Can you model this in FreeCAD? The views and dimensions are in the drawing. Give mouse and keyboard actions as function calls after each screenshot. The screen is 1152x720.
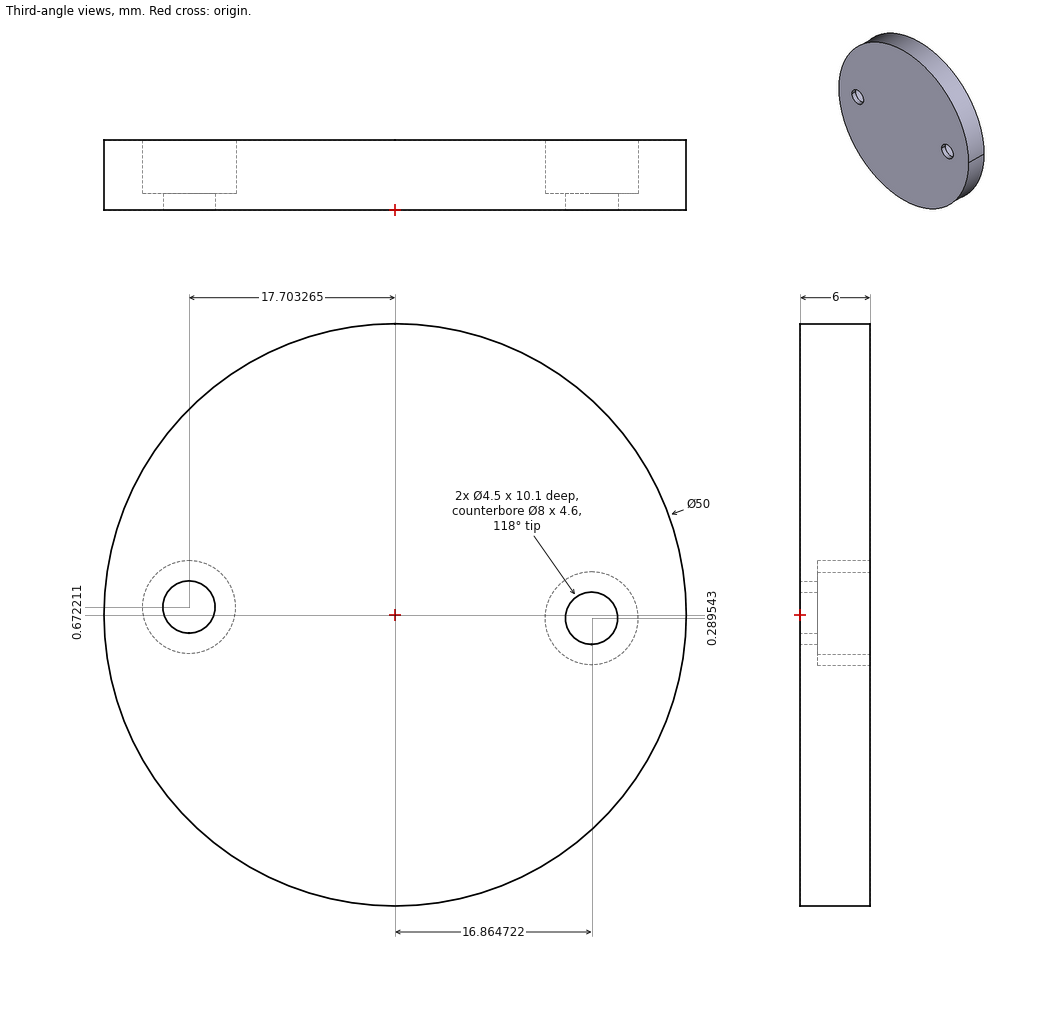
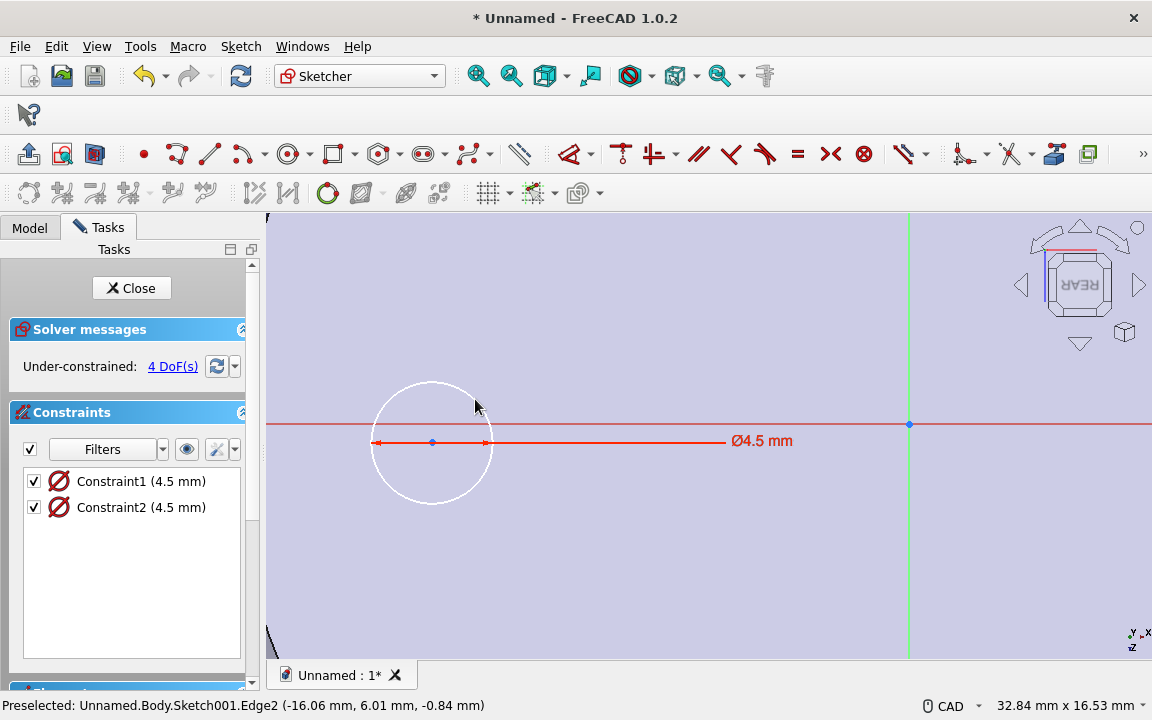
scroll(430, 442, down, 4)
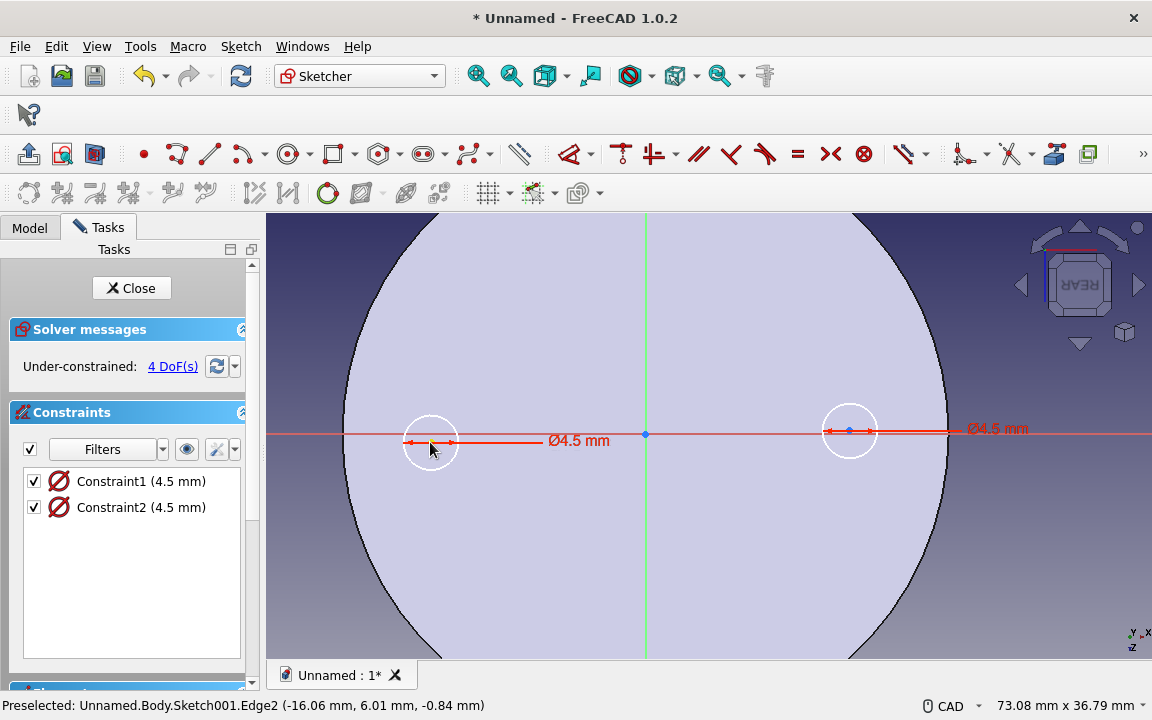
scroll(850, 431, up, 13)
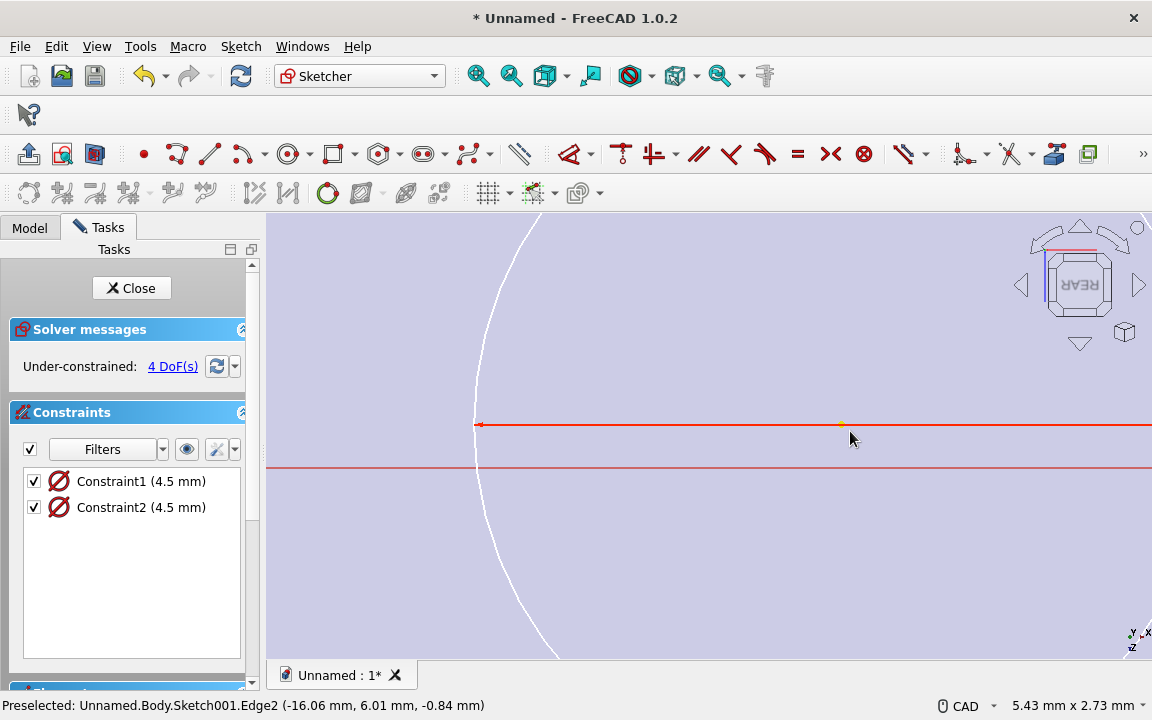
click(841, 425)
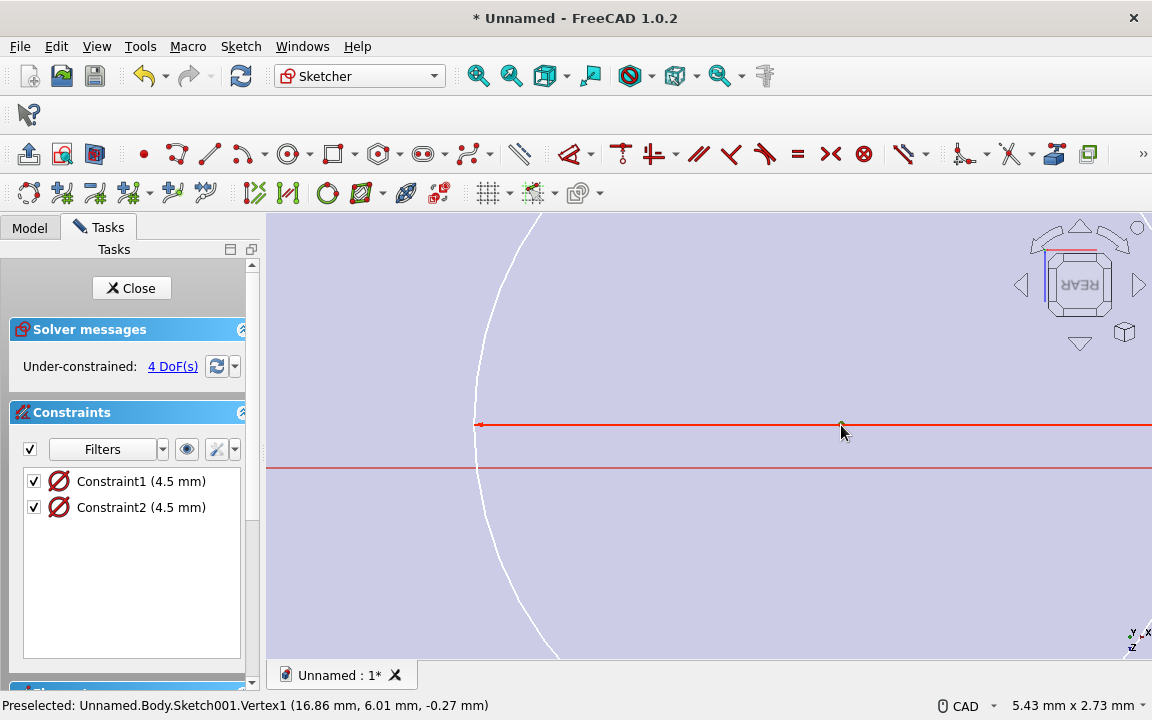
key(i)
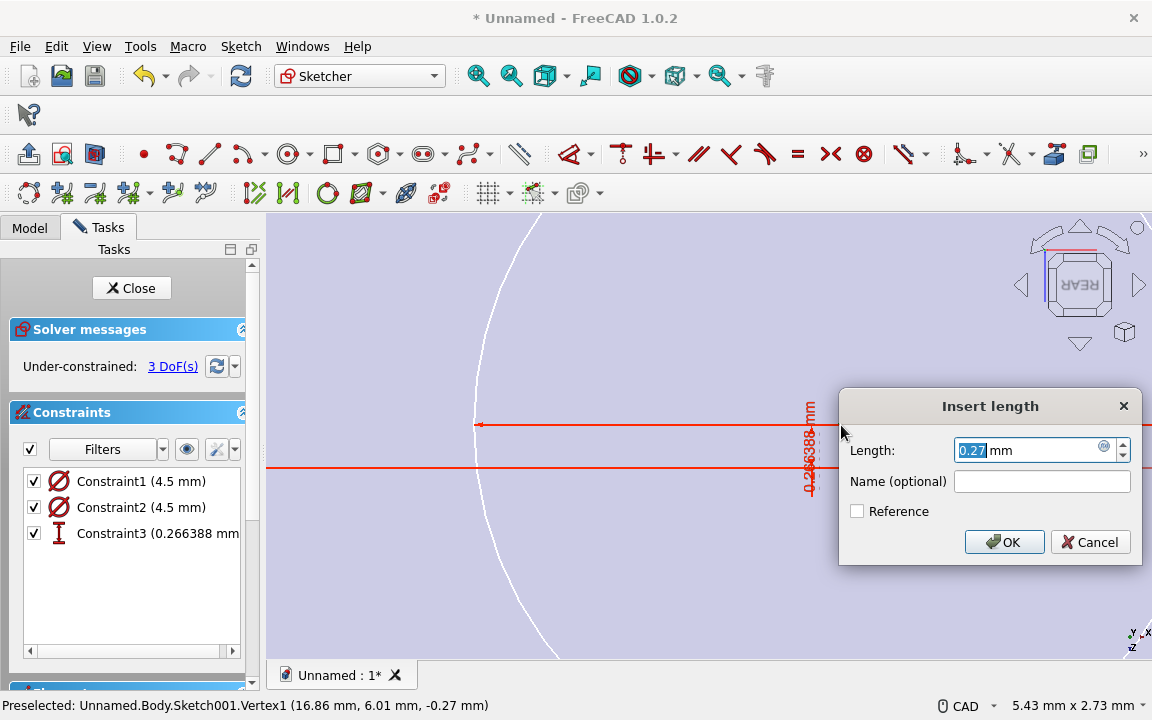
text(0.289543)
key(Return)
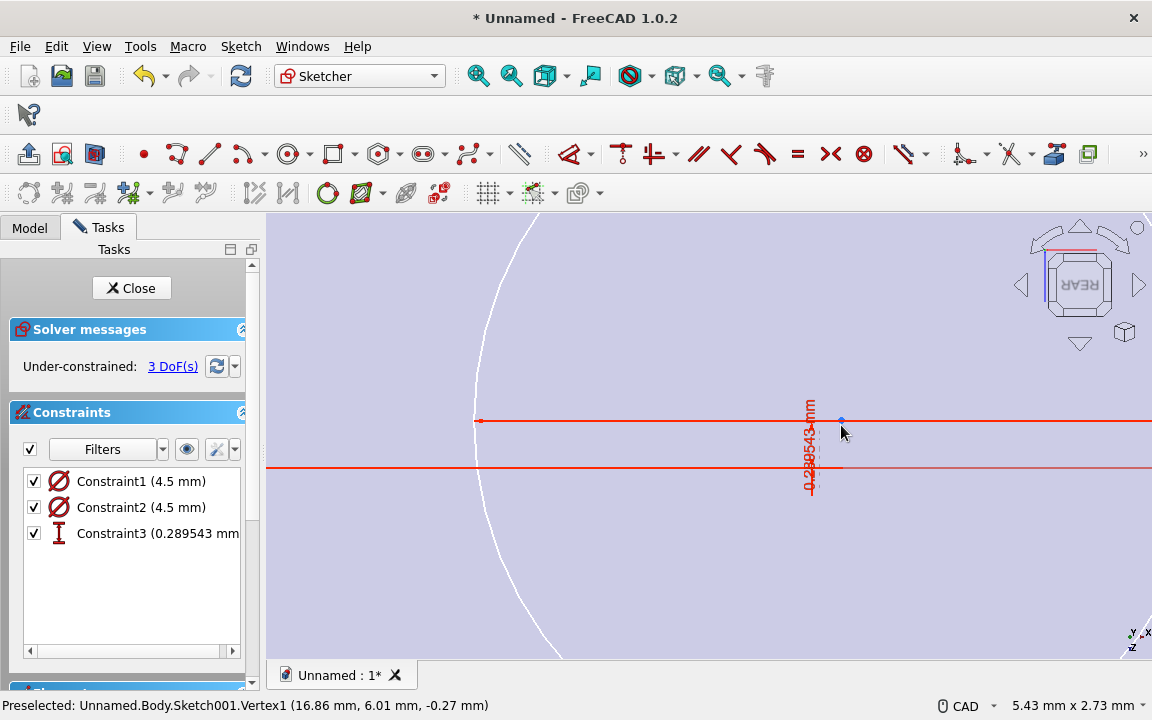
scroll(851, 431, down, 13)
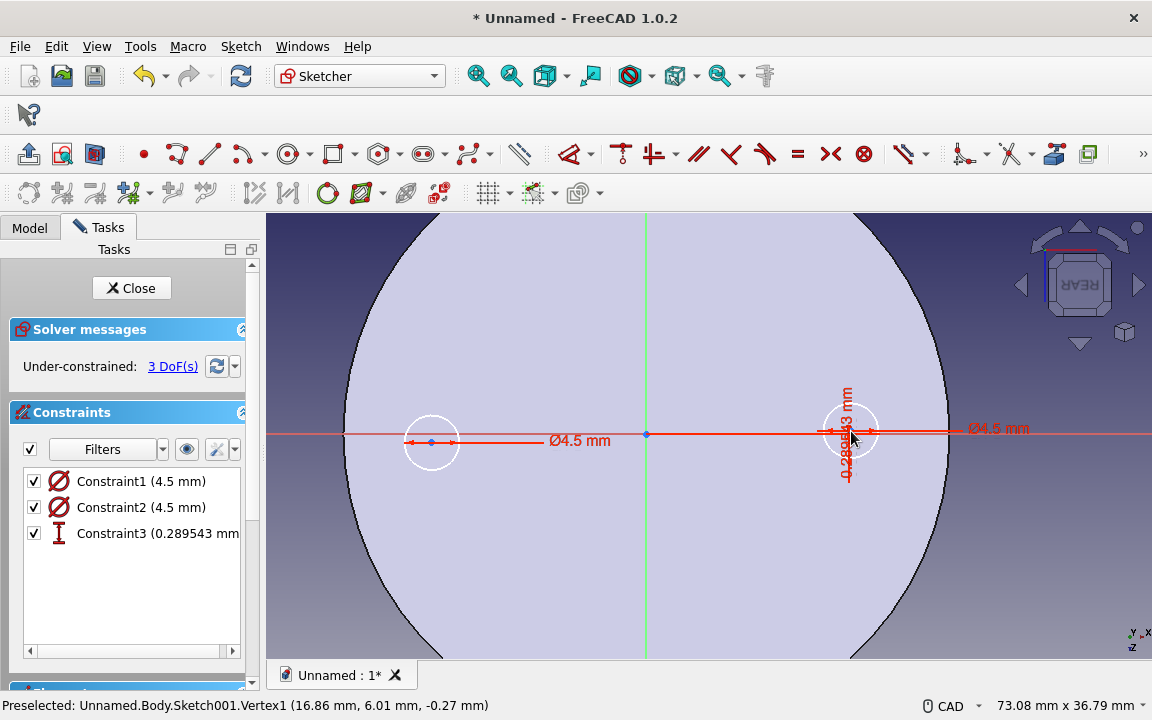
scroll(432, 443, up, 8)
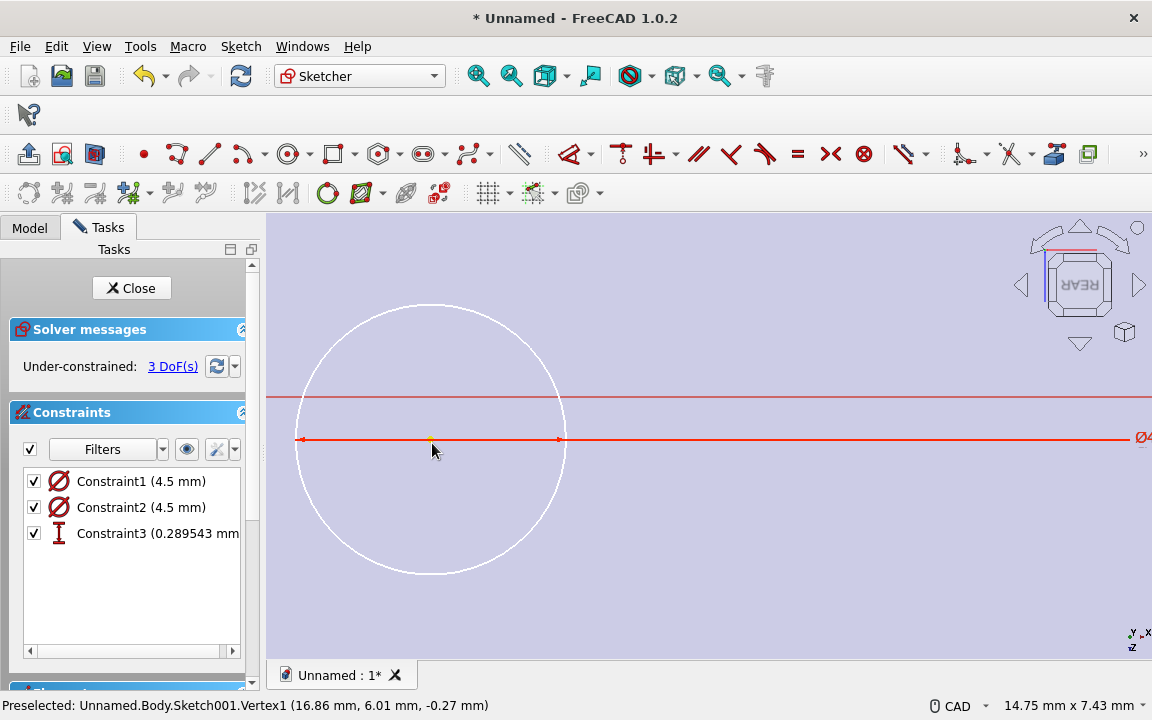
click(431, 440)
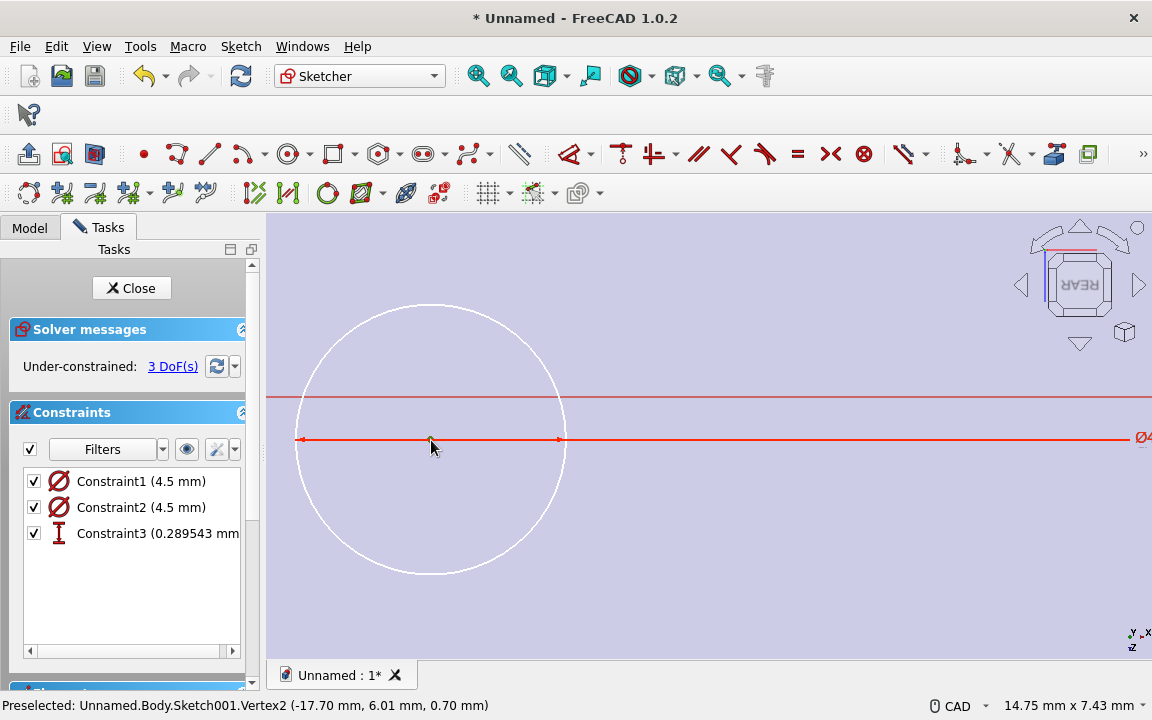
key(i)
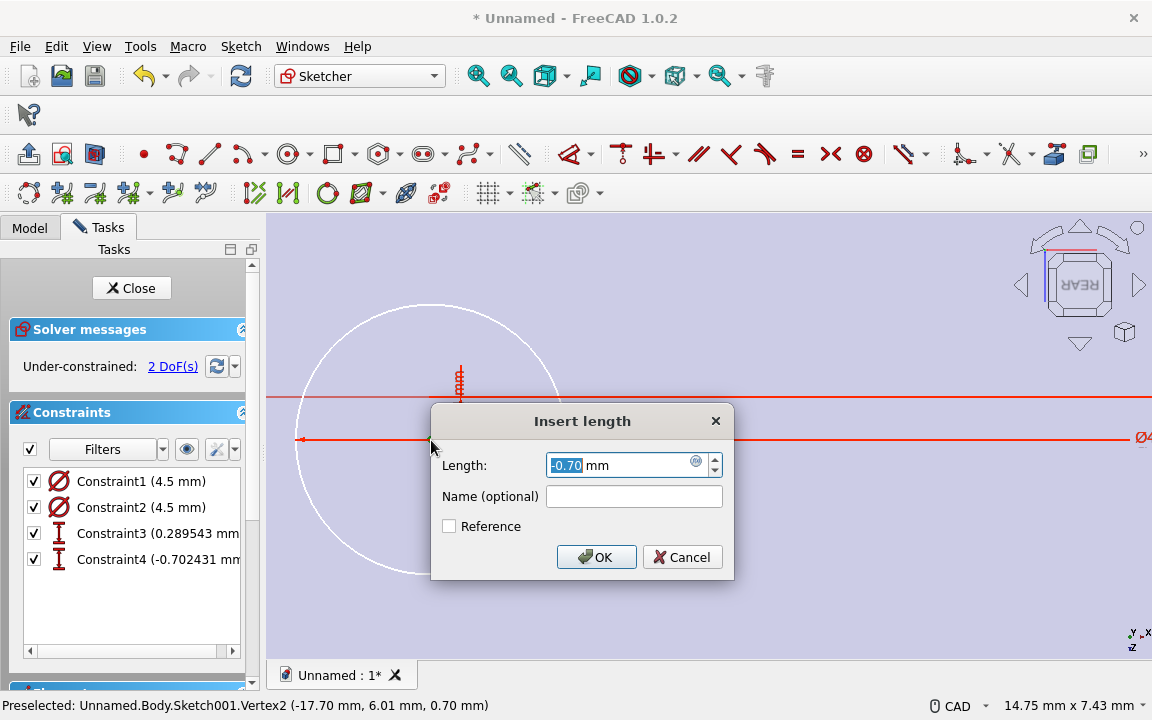
text(-0.672211)
key(Return)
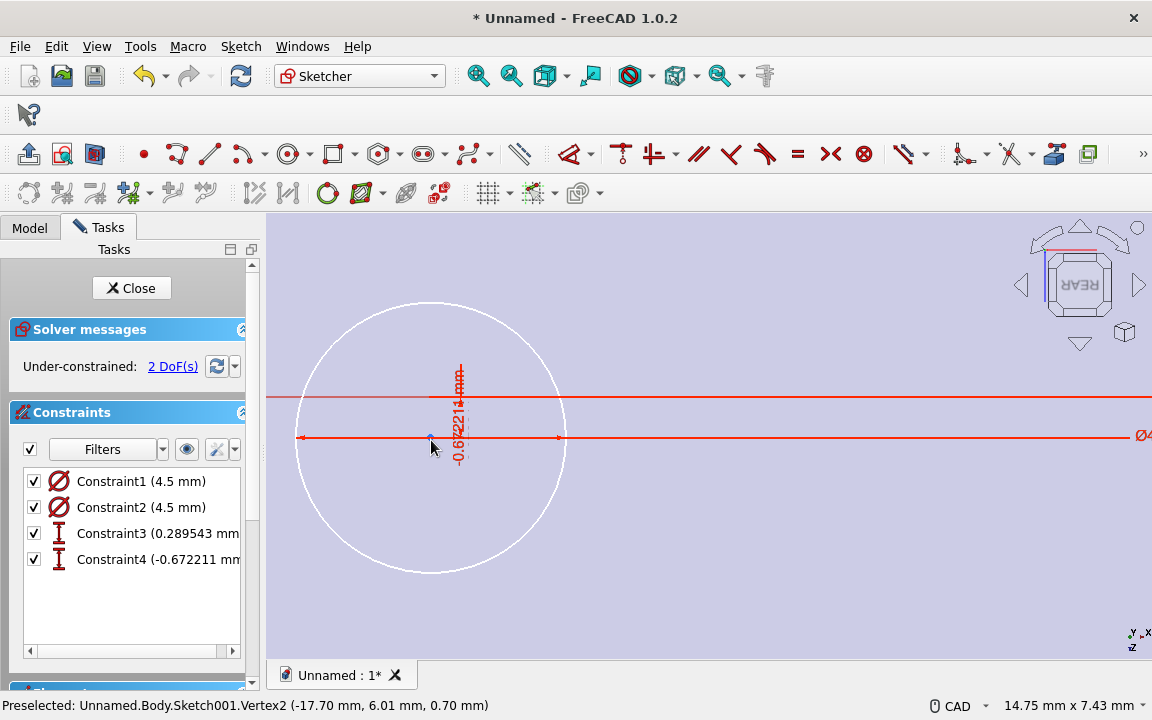
scroll(431, 443, down, 8)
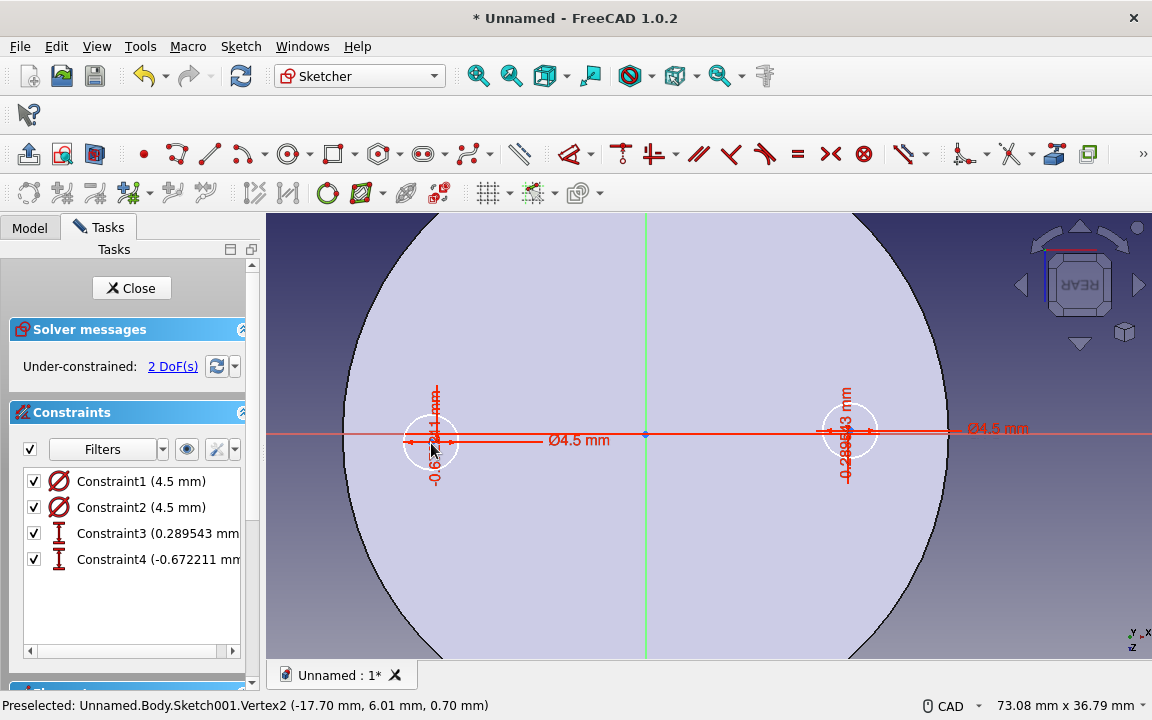
click(850, 431)